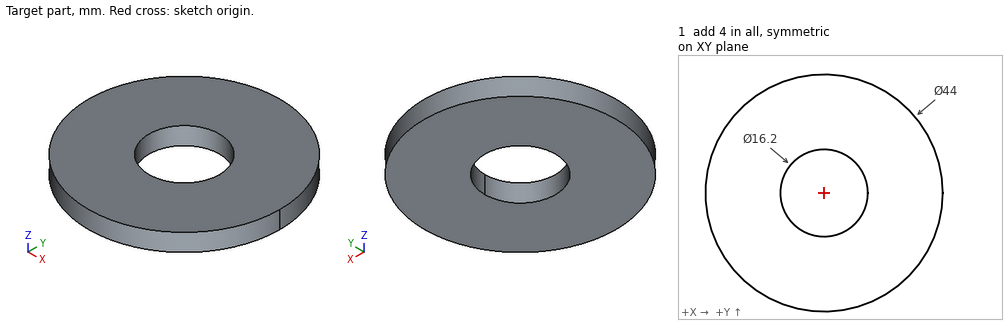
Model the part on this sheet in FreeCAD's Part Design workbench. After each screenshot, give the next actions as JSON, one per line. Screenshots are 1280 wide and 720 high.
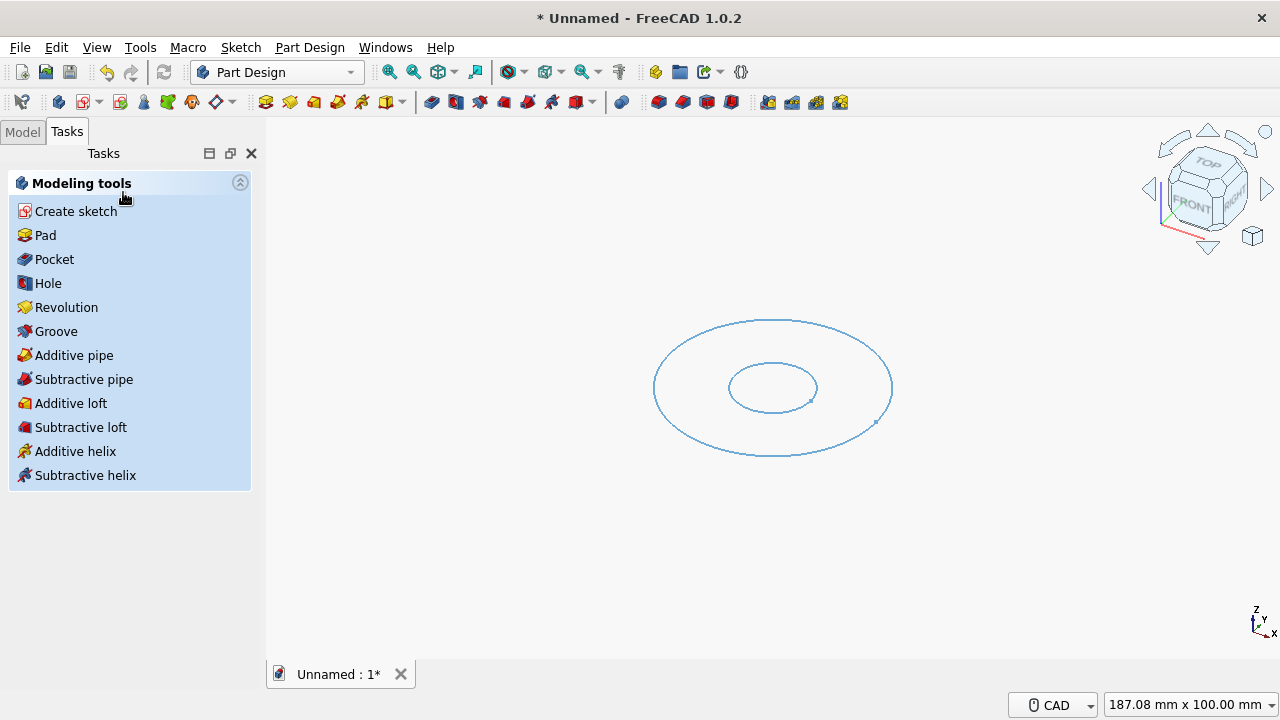
{"action": "left_click", "coordinate": [266, 102]}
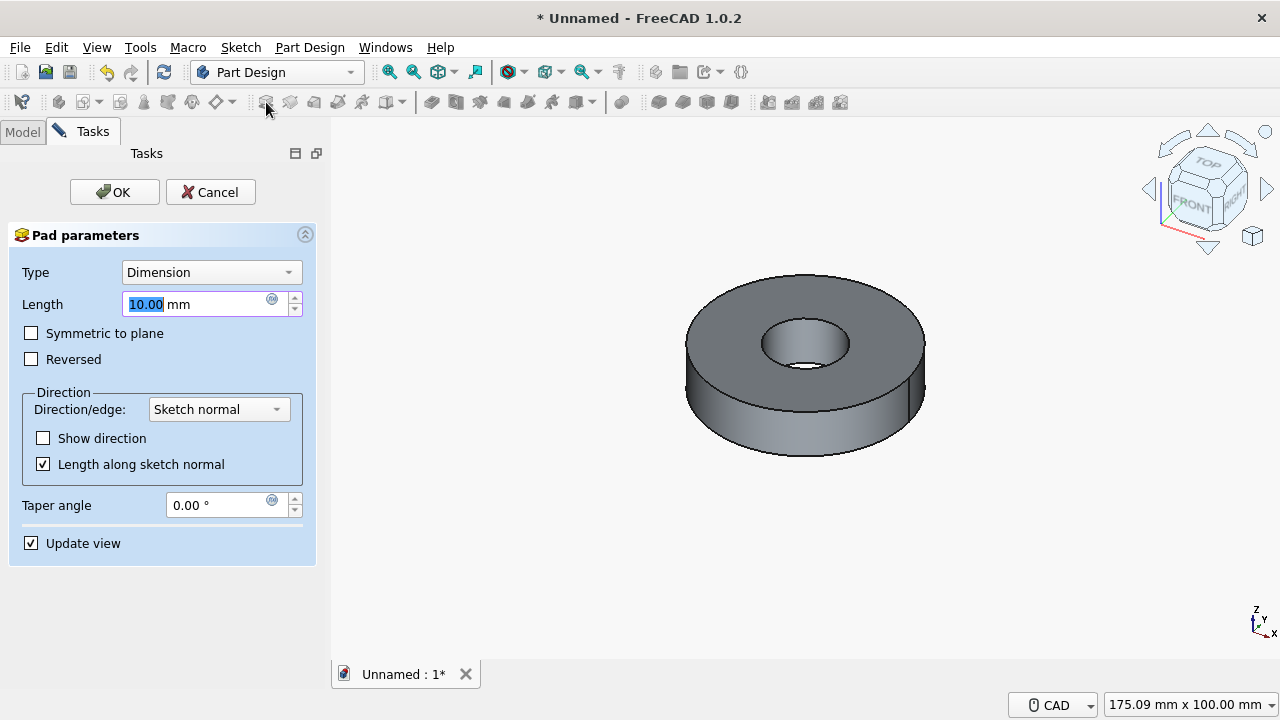
{"action": "type", "text": "4"}
{"action": "key", "text": "Tab"}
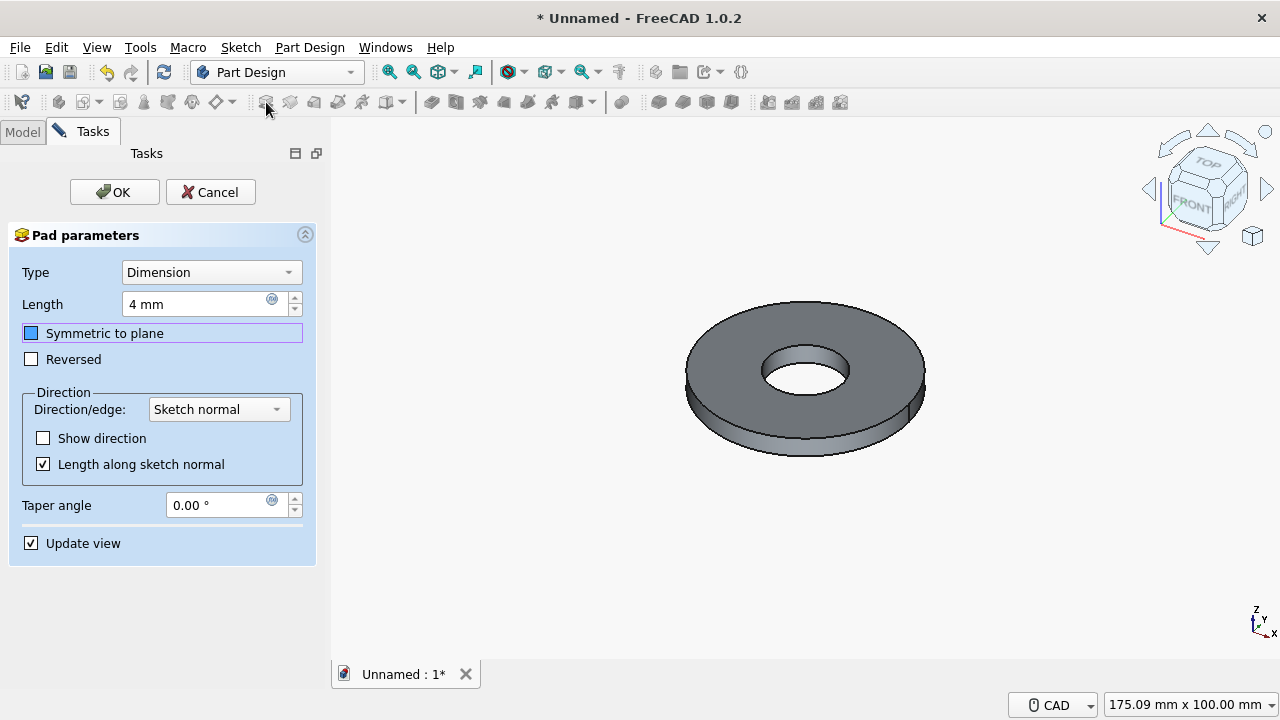
{"action": "left_click", "coordinate": [30, 333]}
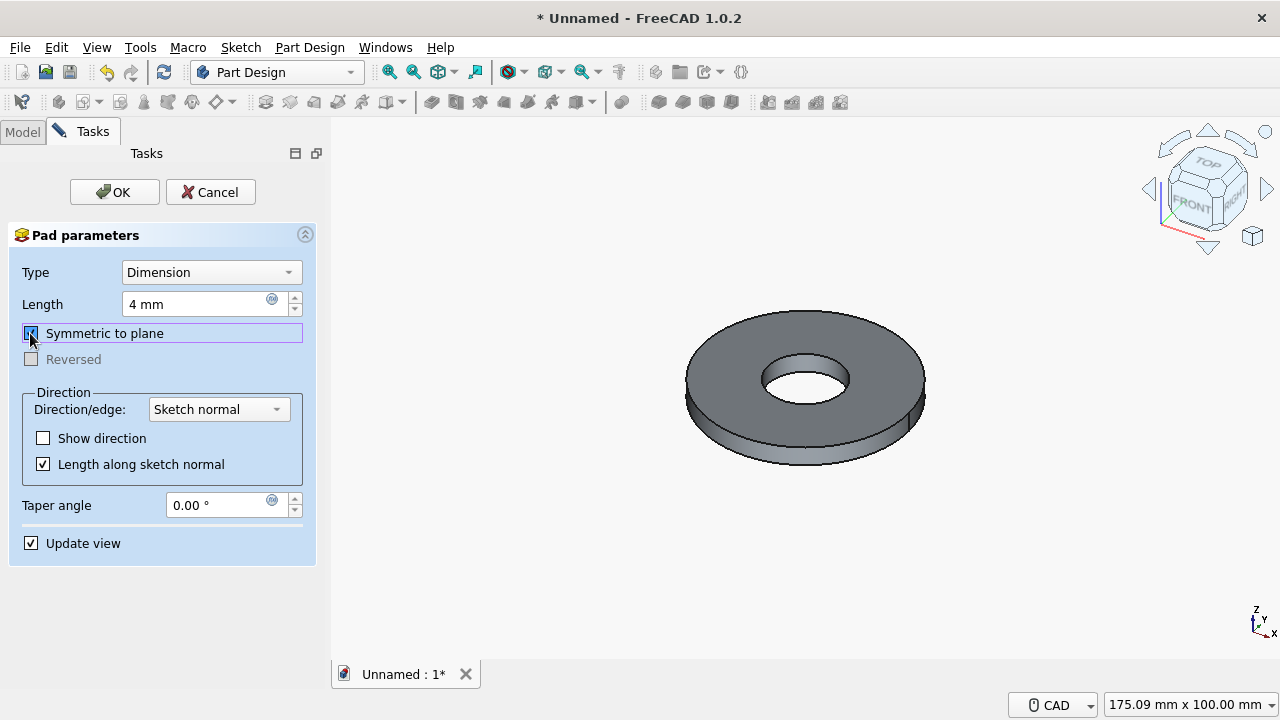
{"action": "left_click", "coordinate": [115, 192]}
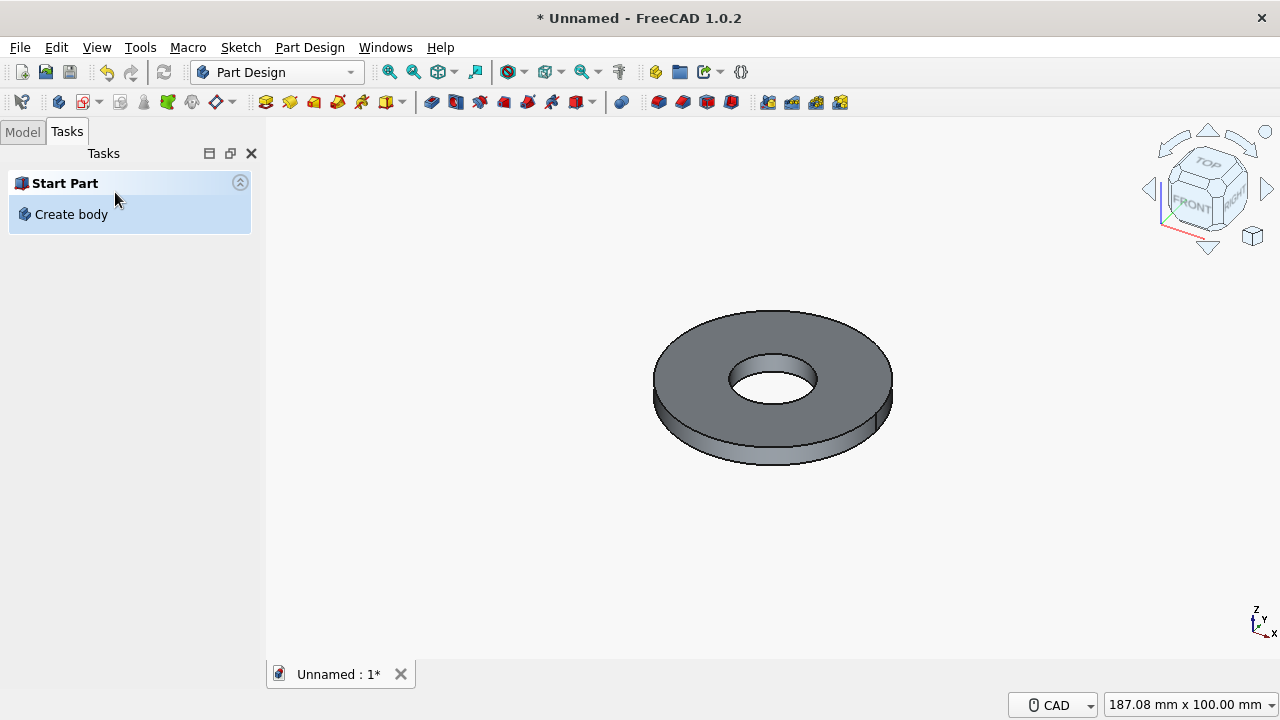
{"action": "key", "text": "0"}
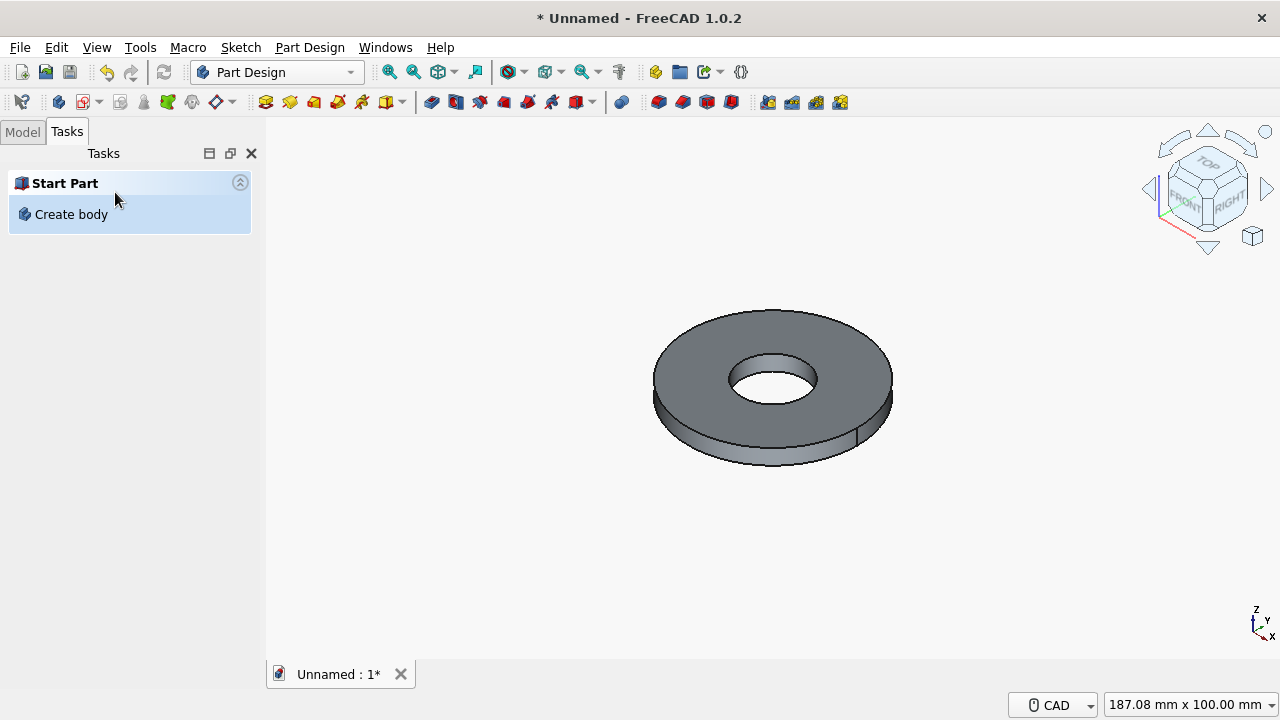
{"action": "left_click", "coordinate": [390, 72]}